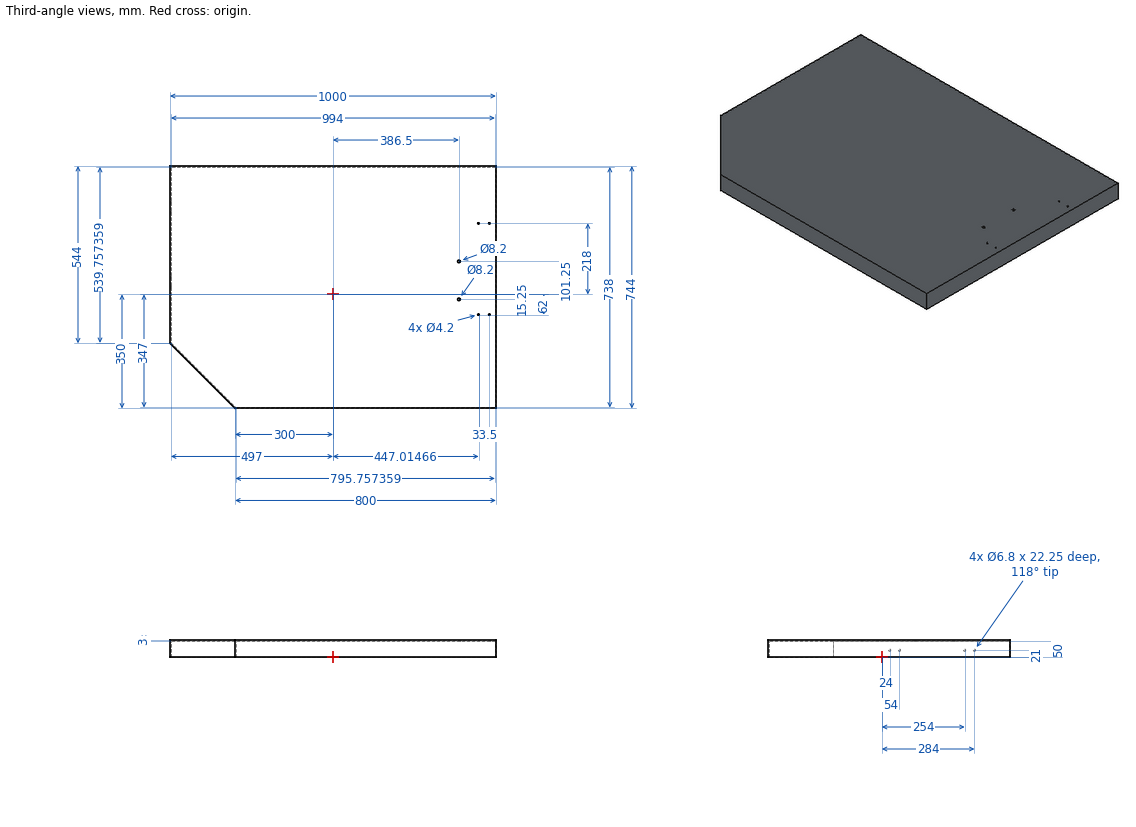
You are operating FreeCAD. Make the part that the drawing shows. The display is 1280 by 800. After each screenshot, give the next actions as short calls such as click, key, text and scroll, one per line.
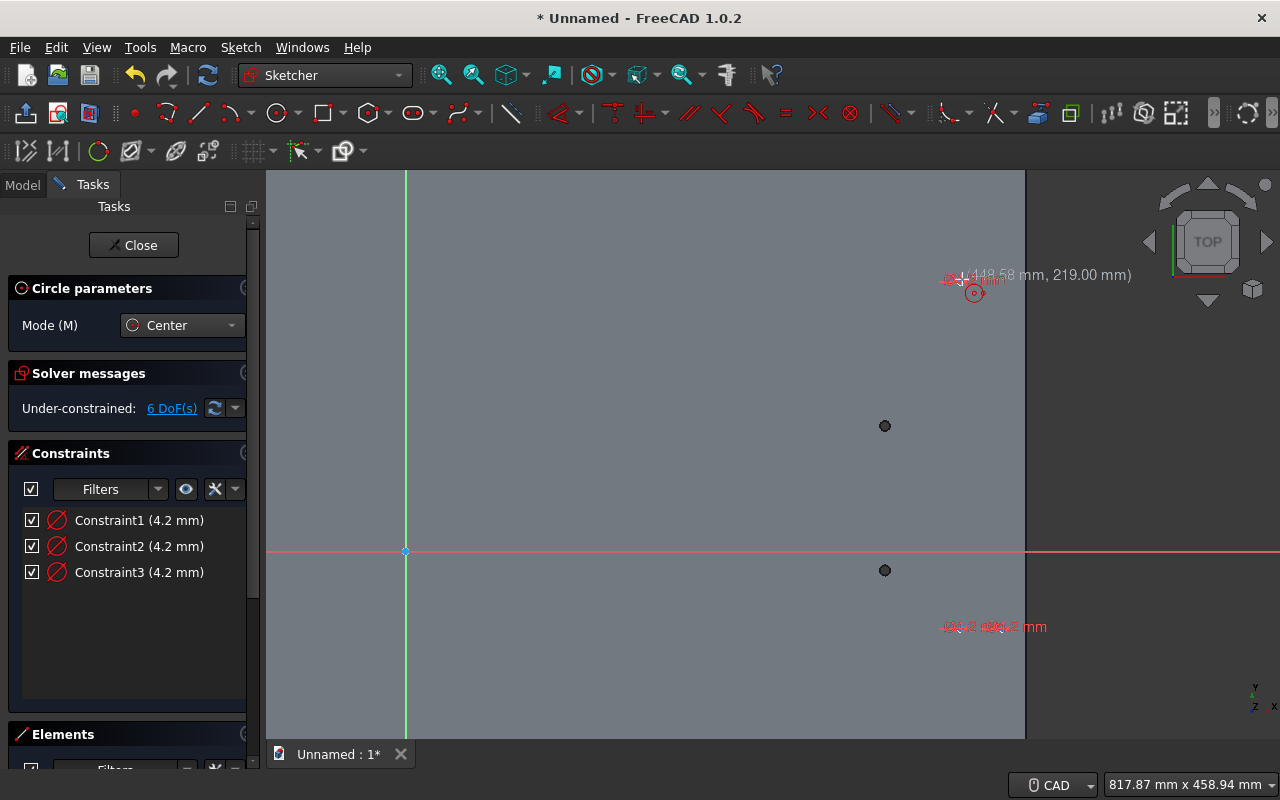
scroll(1002, 281, up, 11)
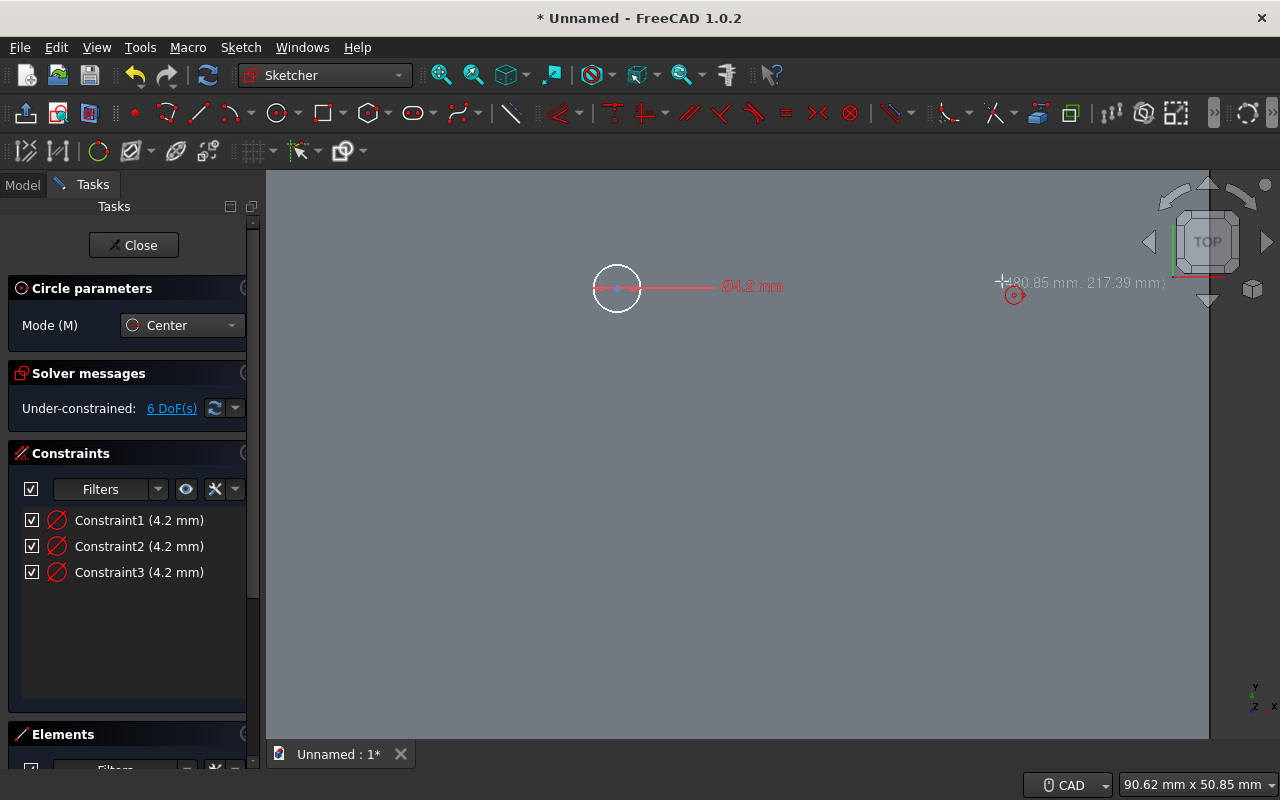
scroll(1002, 281, down, 11)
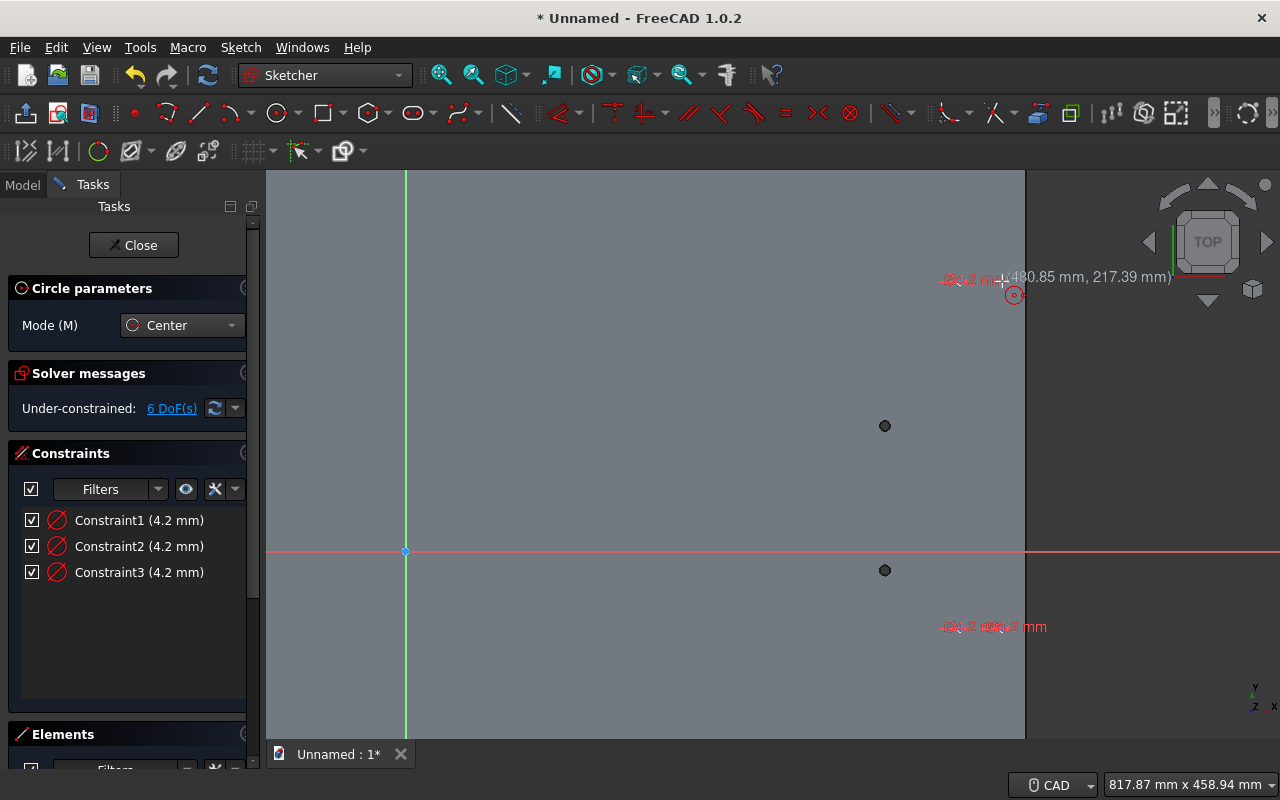
click(1002, 281)
move(1003, 279)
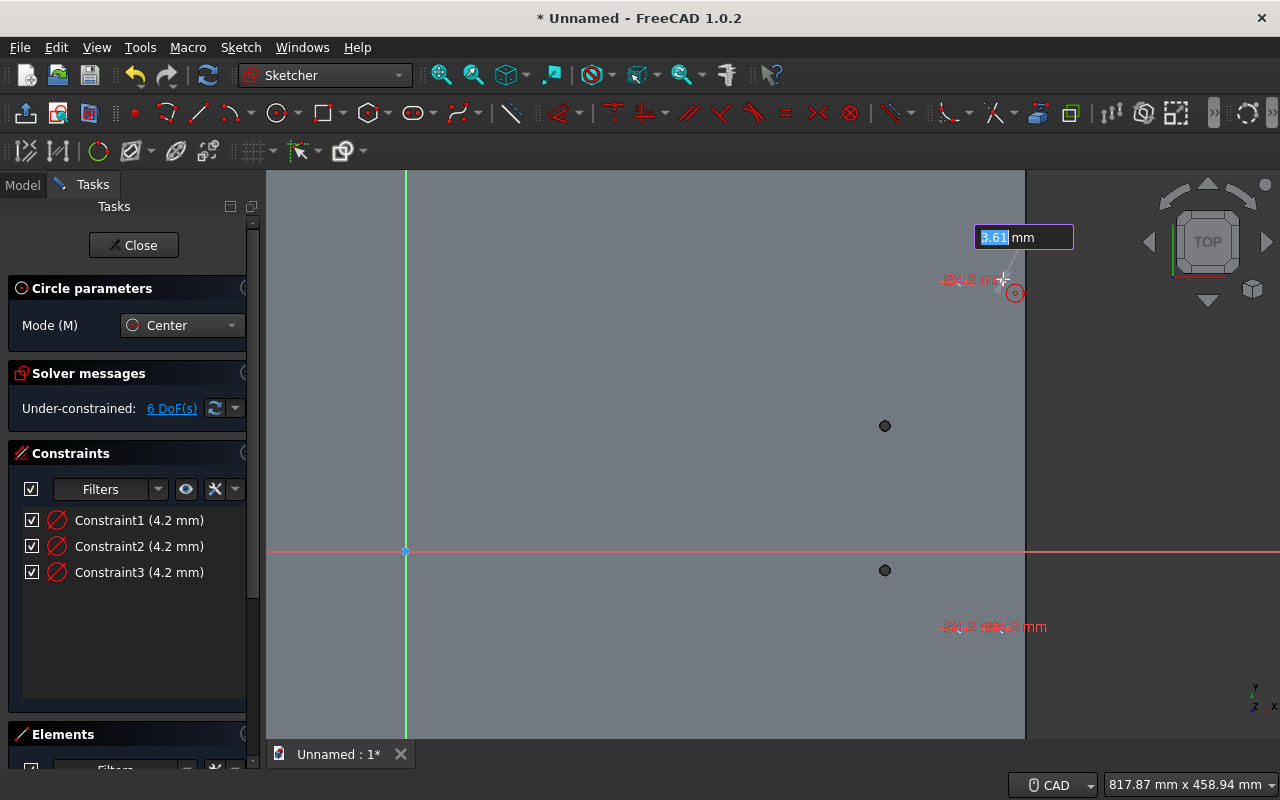
text(4.2)
key(Return)
key(Escape)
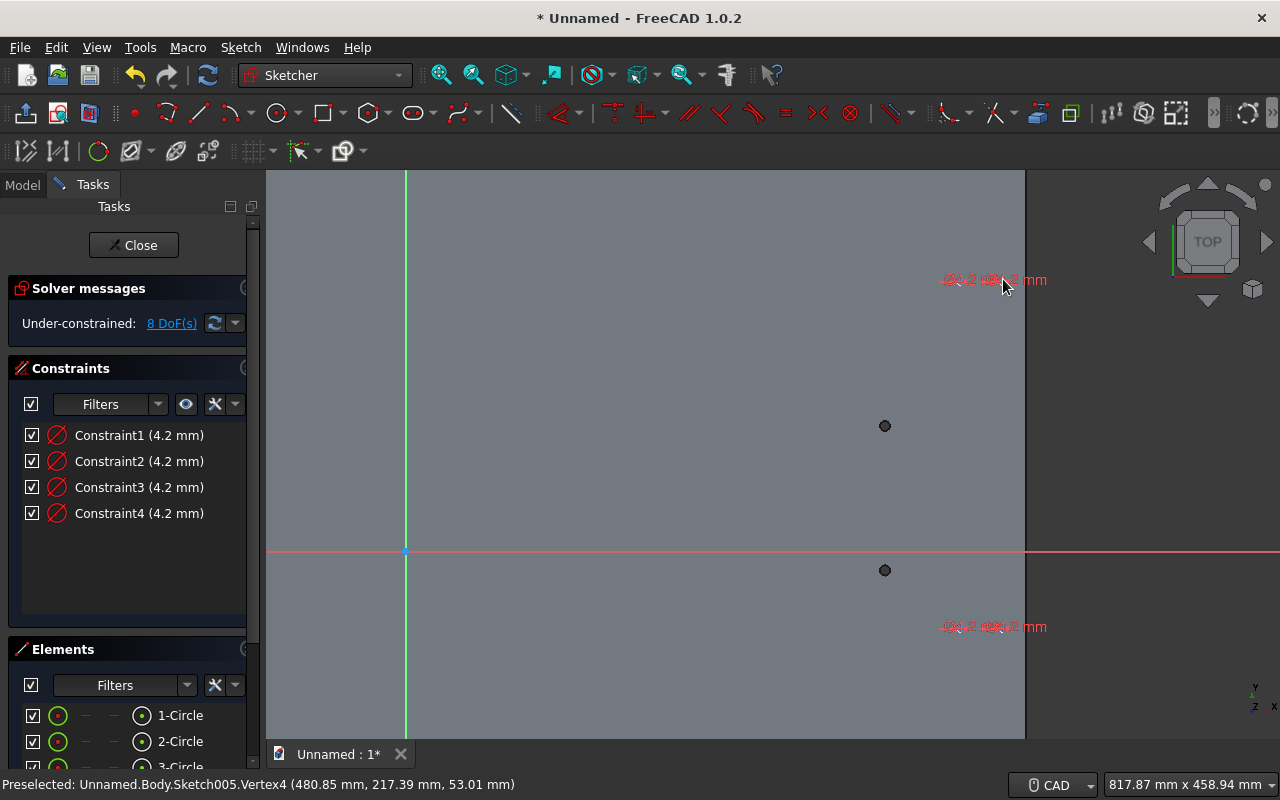
click(558, 114)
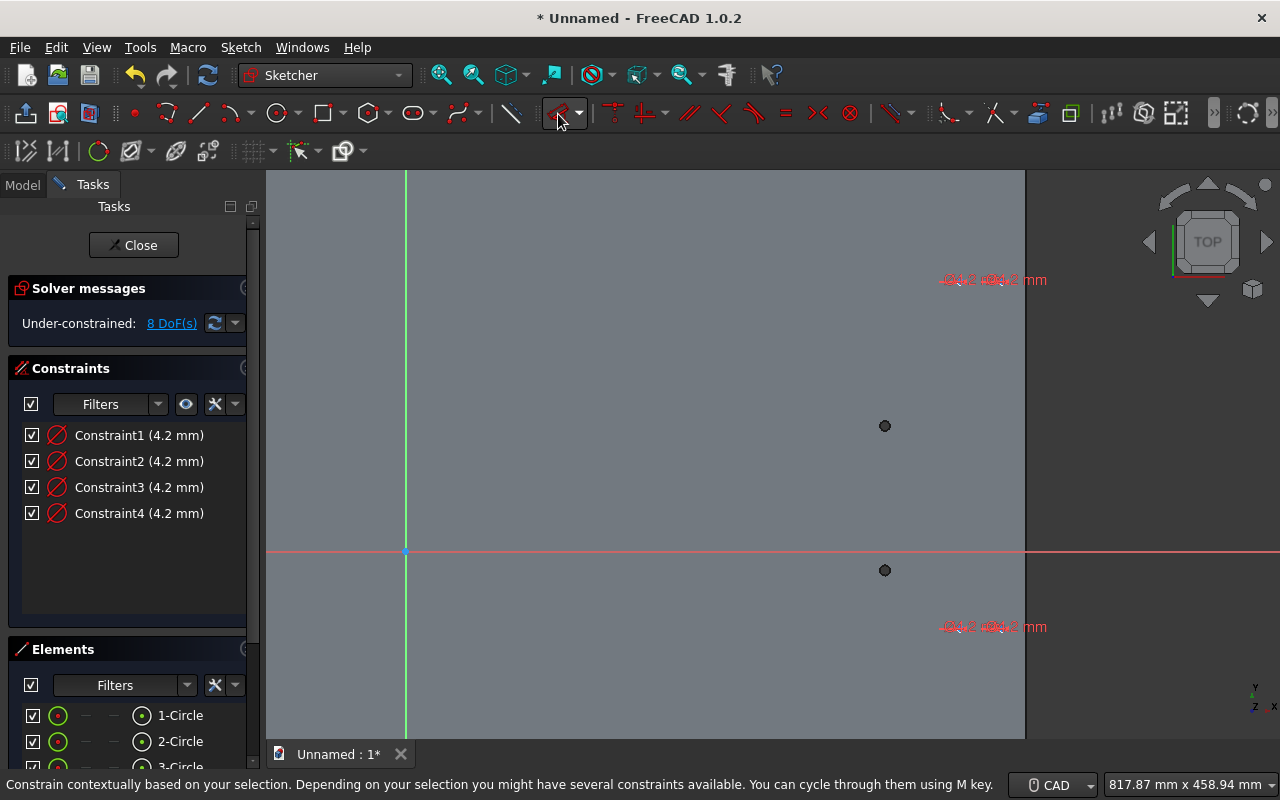
click(960, 629)
click(372, 590)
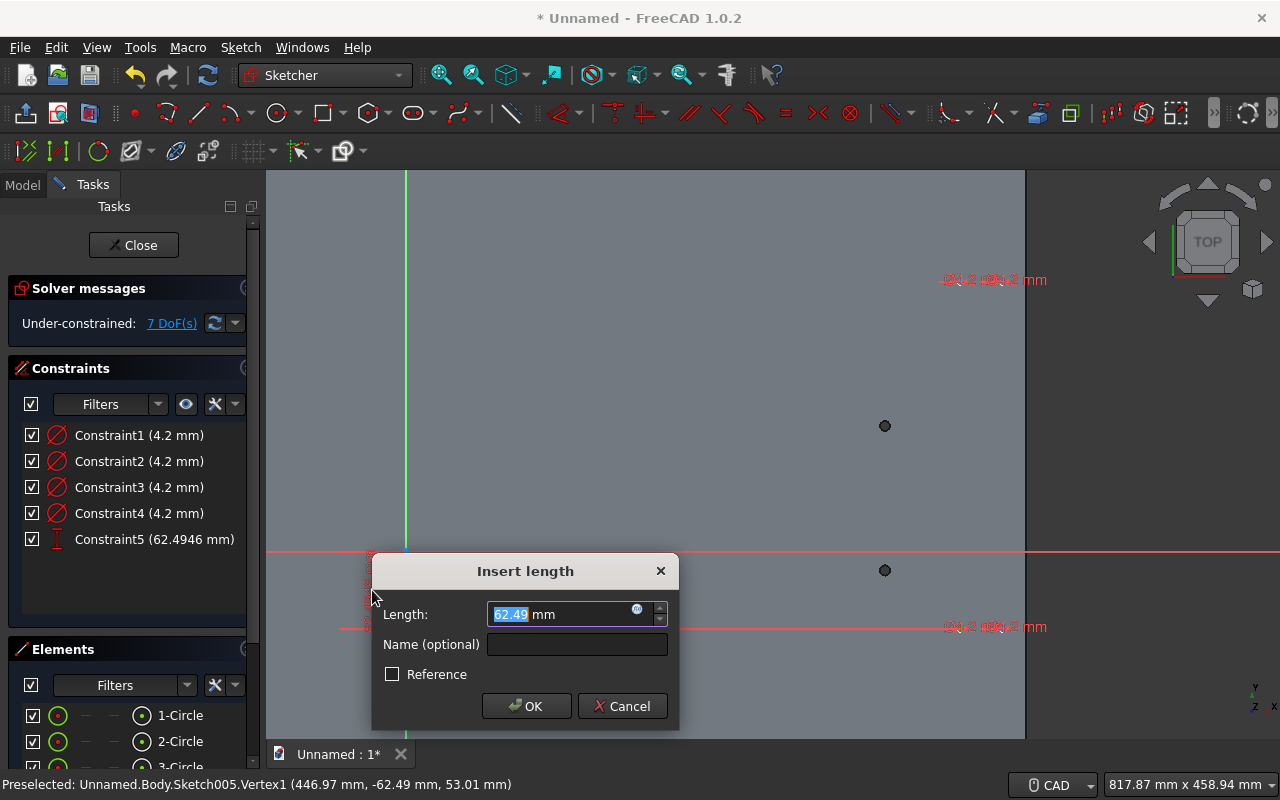
text(62)
key(Return)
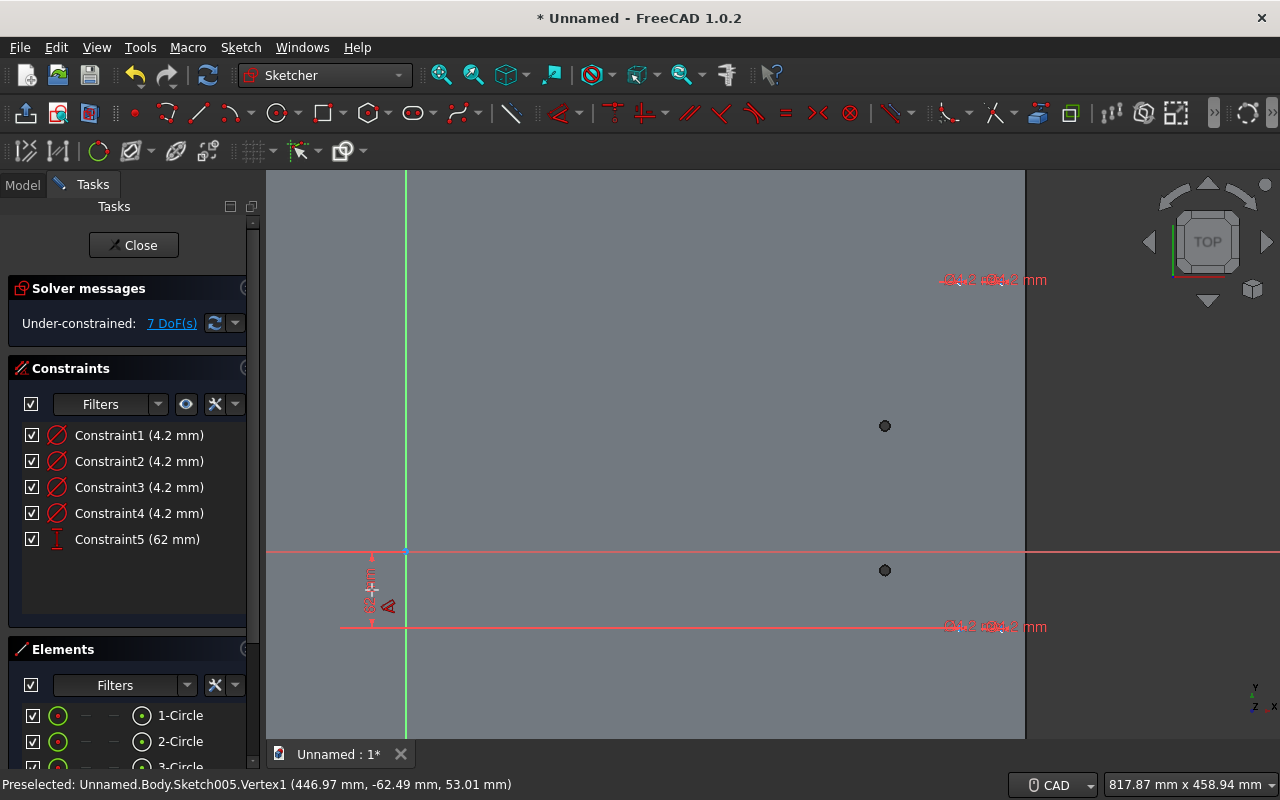
click(1002, 629)
click(372, 617)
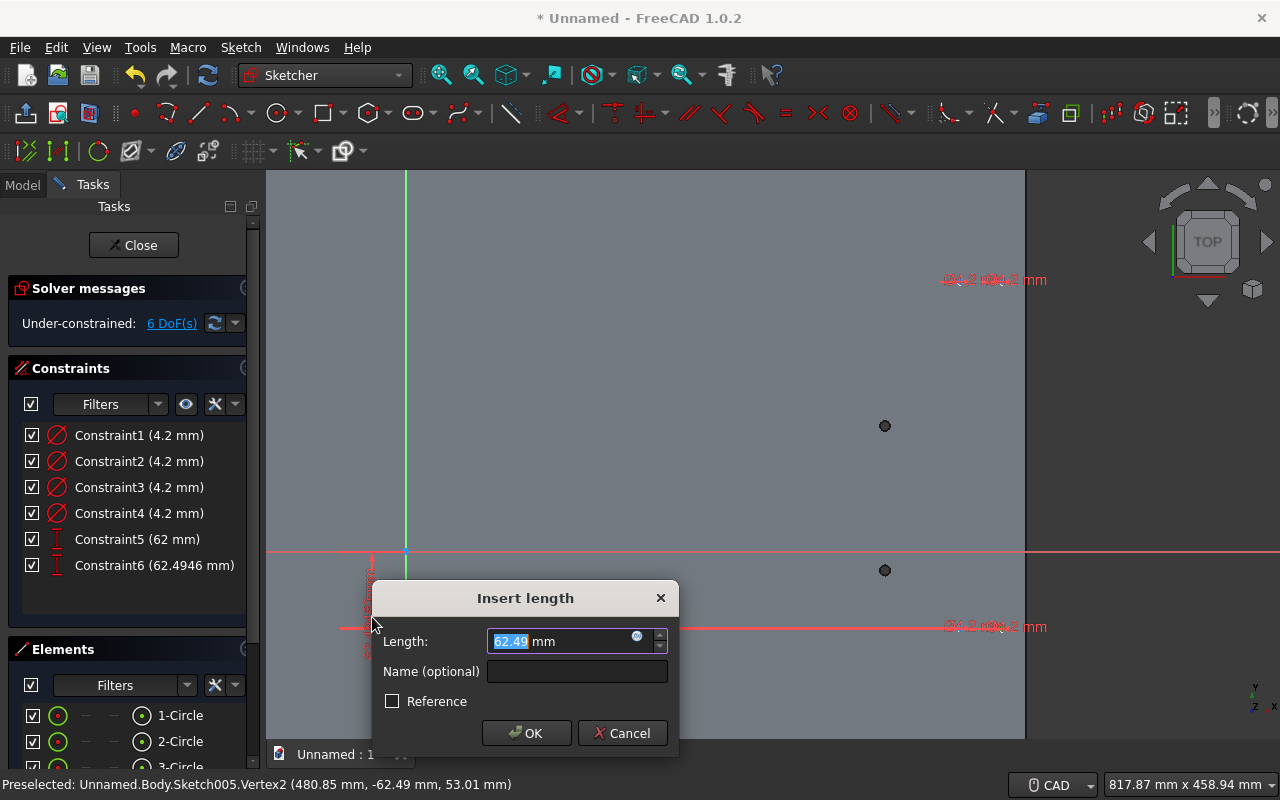
text(62)
key(Return)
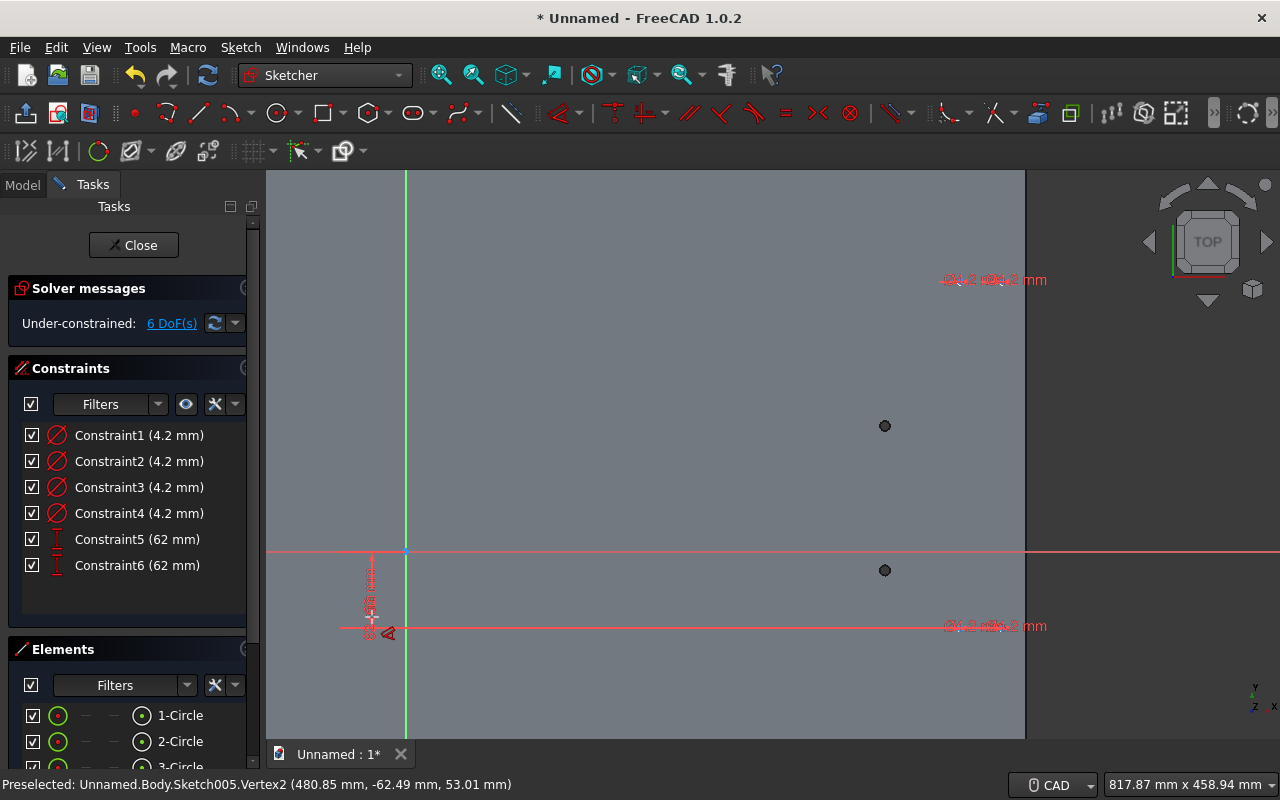
click(960, 282)
click(372, 417)